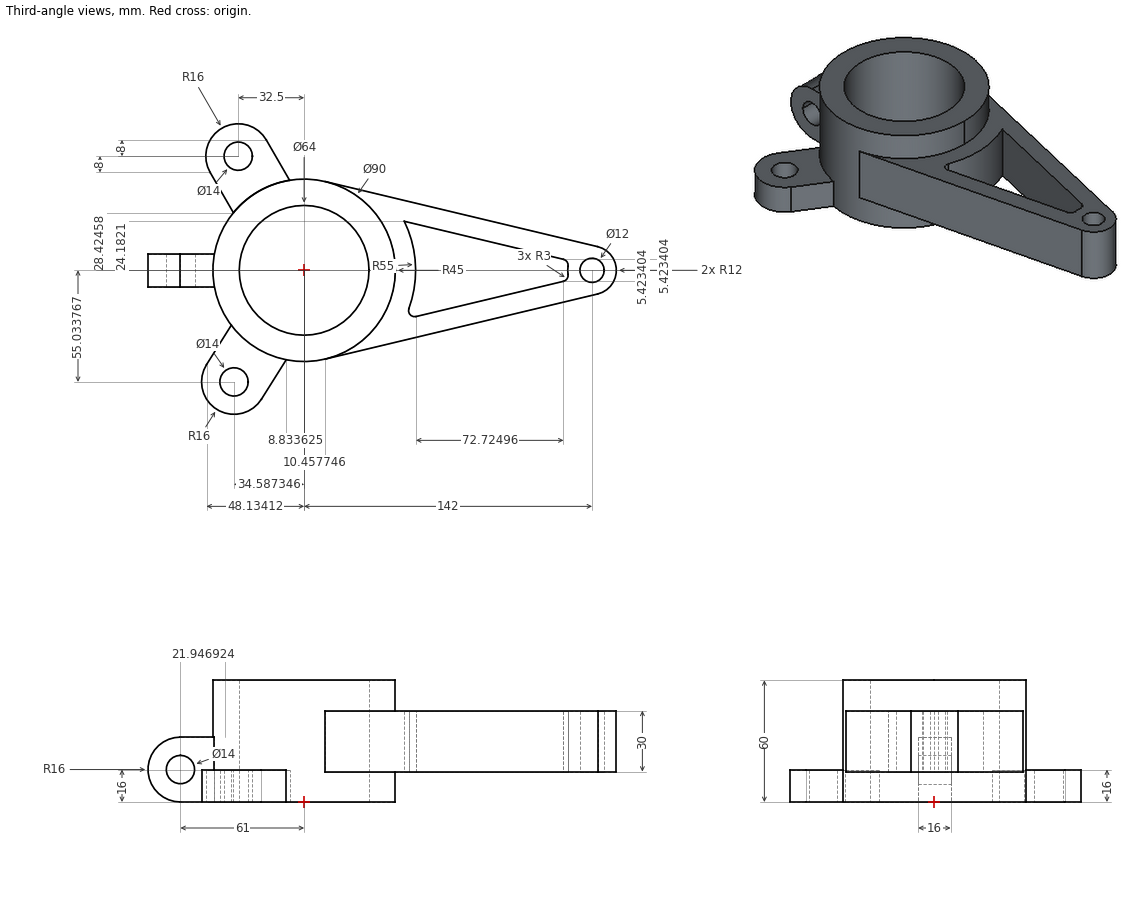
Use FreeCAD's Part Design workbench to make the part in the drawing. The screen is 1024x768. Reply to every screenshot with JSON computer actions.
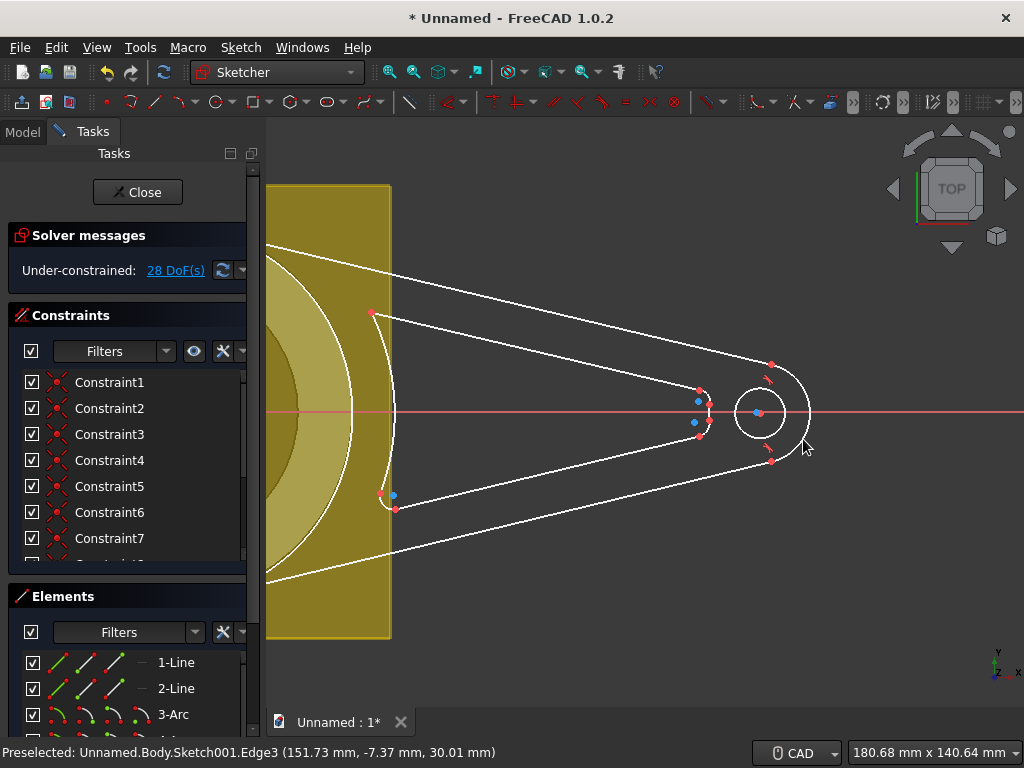
{"action": "left_click", "coordinate": [608, 458]}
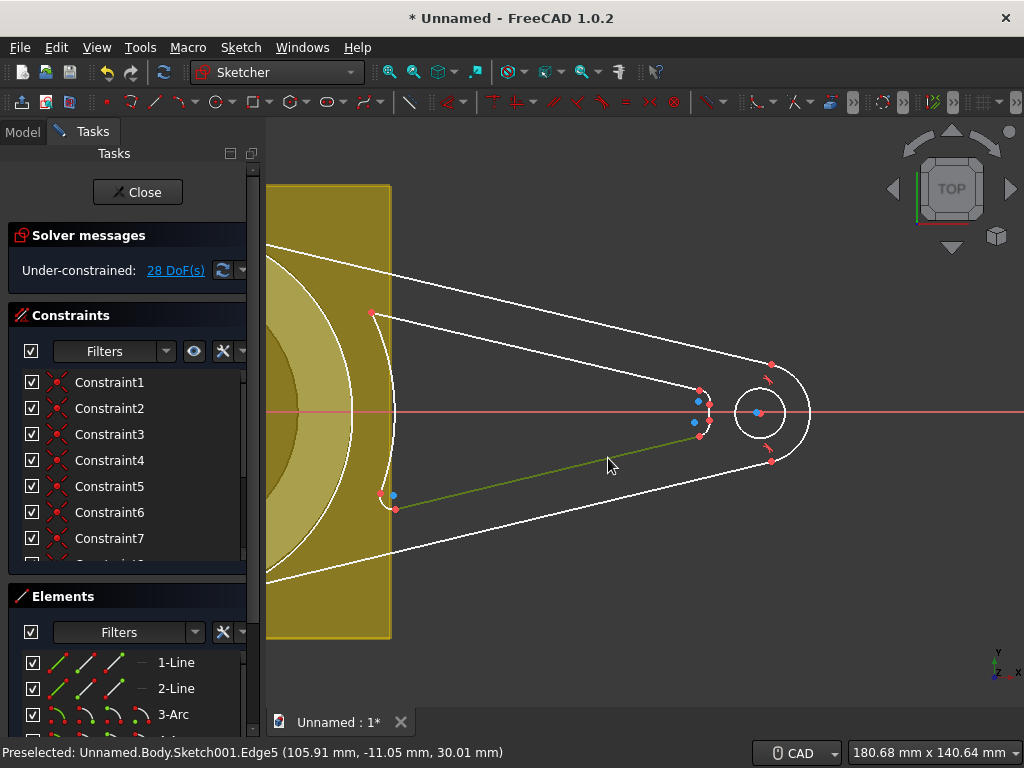
{"action": "left_click", "coordinate": [384, 505]}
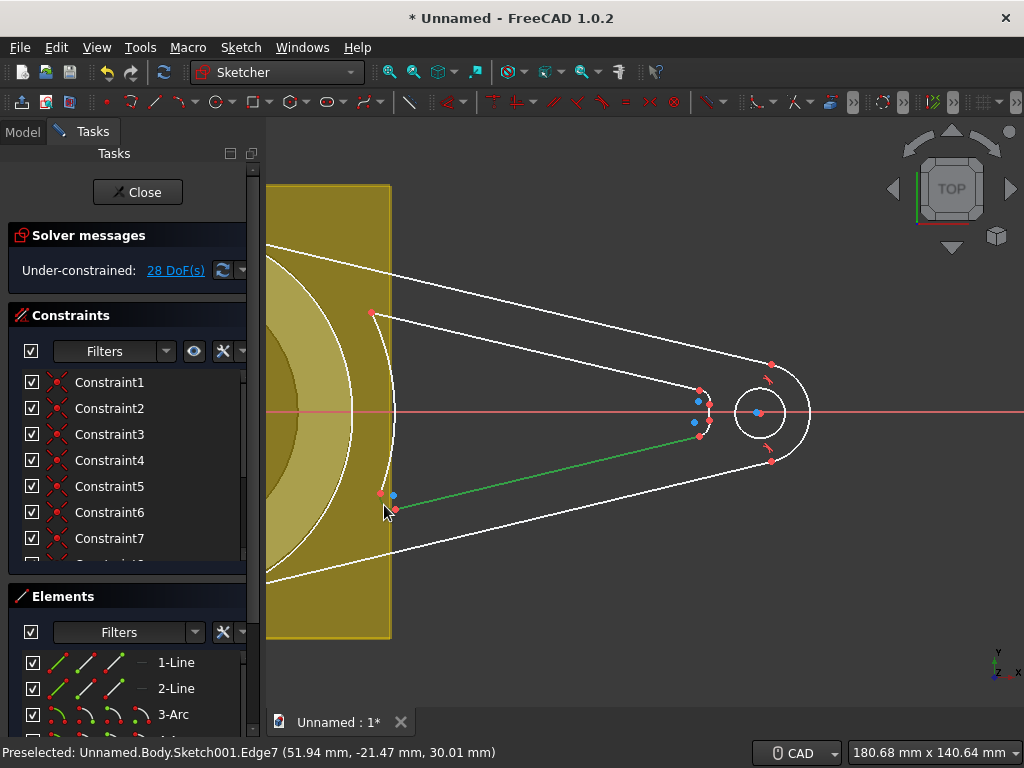
{"action": "key", "text": "t"}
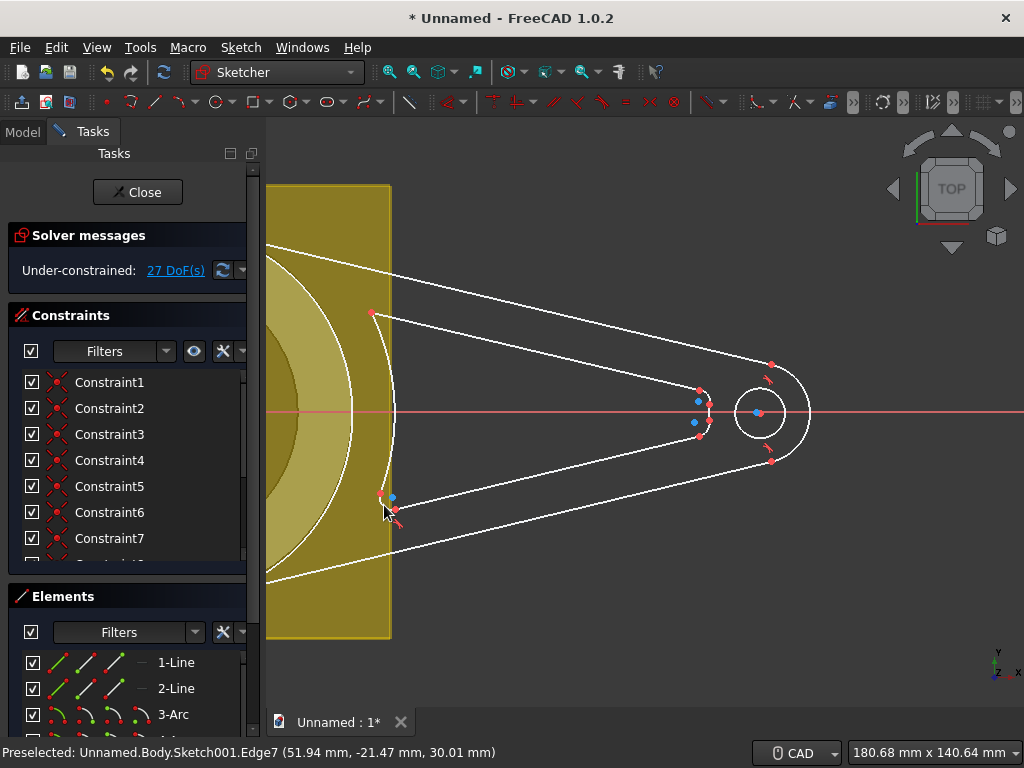
{"action": "left_click", "coordinate": [608, 458]}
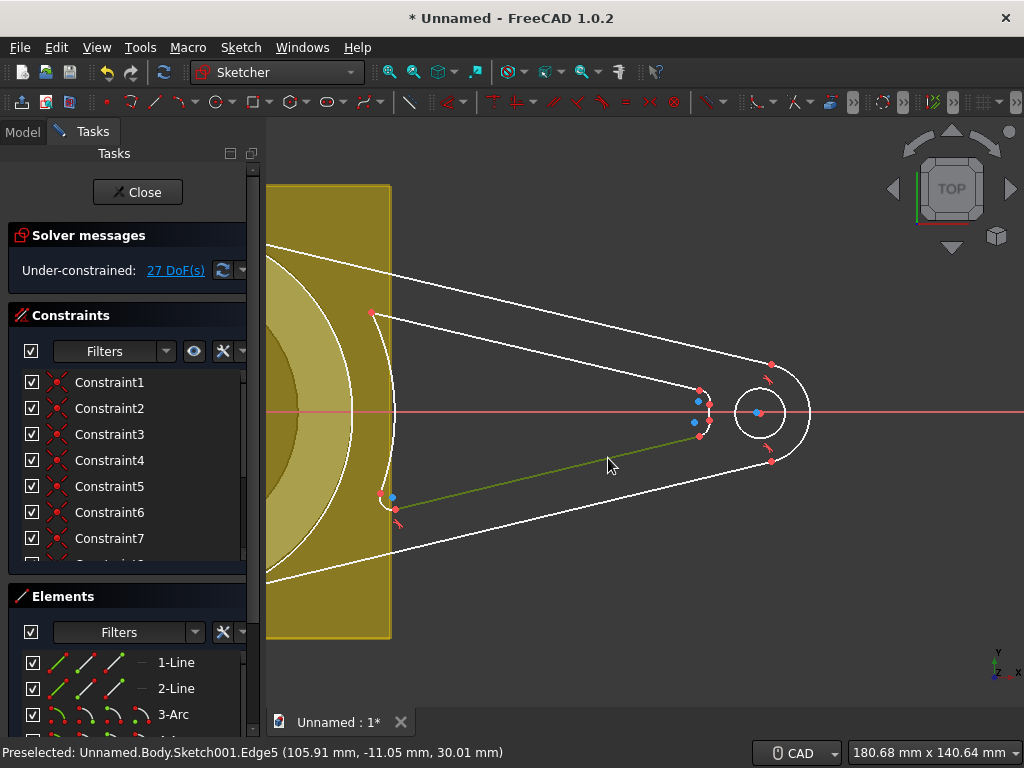
{"action": "scroll", "coordinate": [707, 430], "scroll_direction": "up", "scroll_amount": 2}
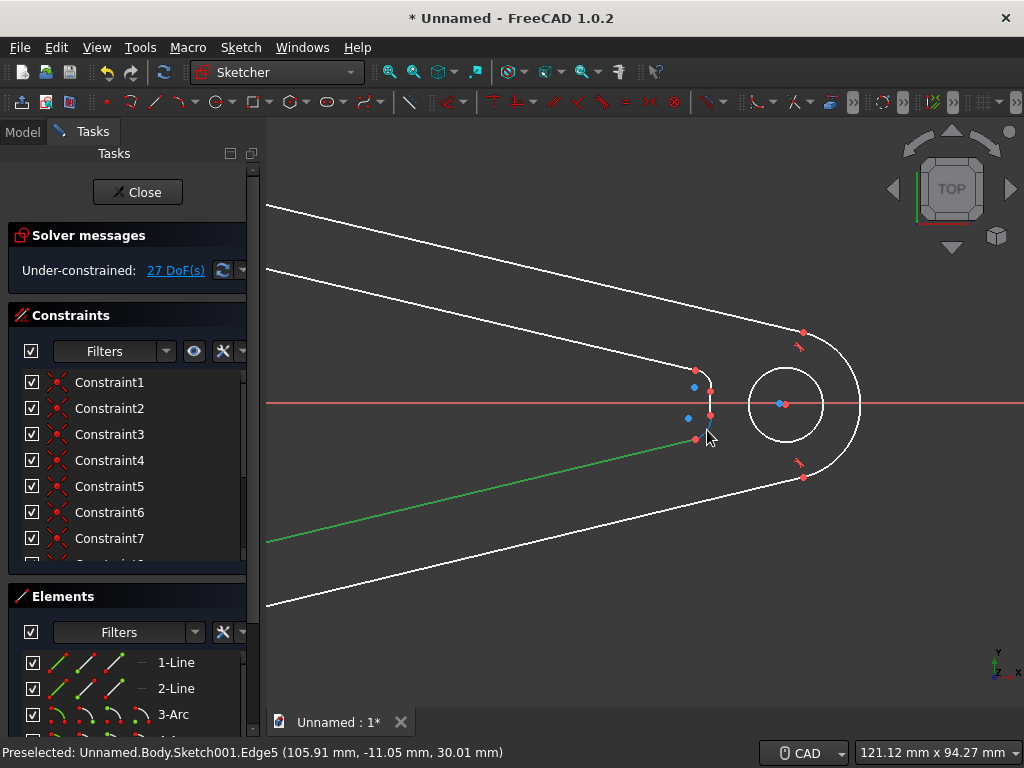
{"action": "left_click", "coordinate": [707, 430]}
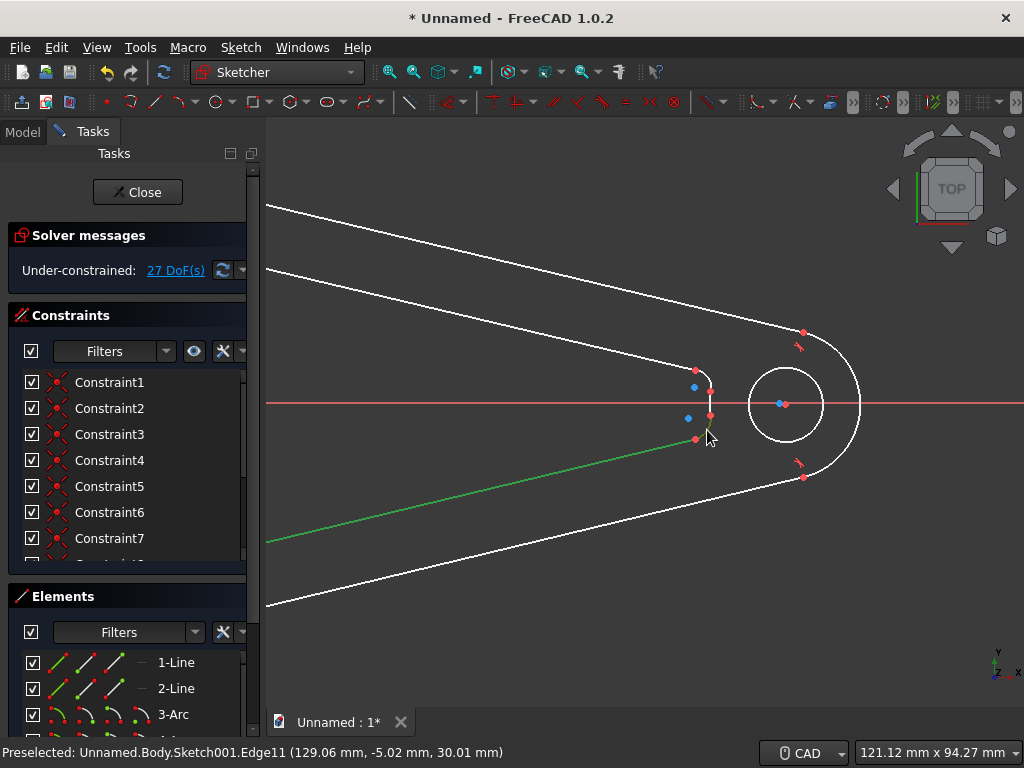
{"action": "key", "text": "t"}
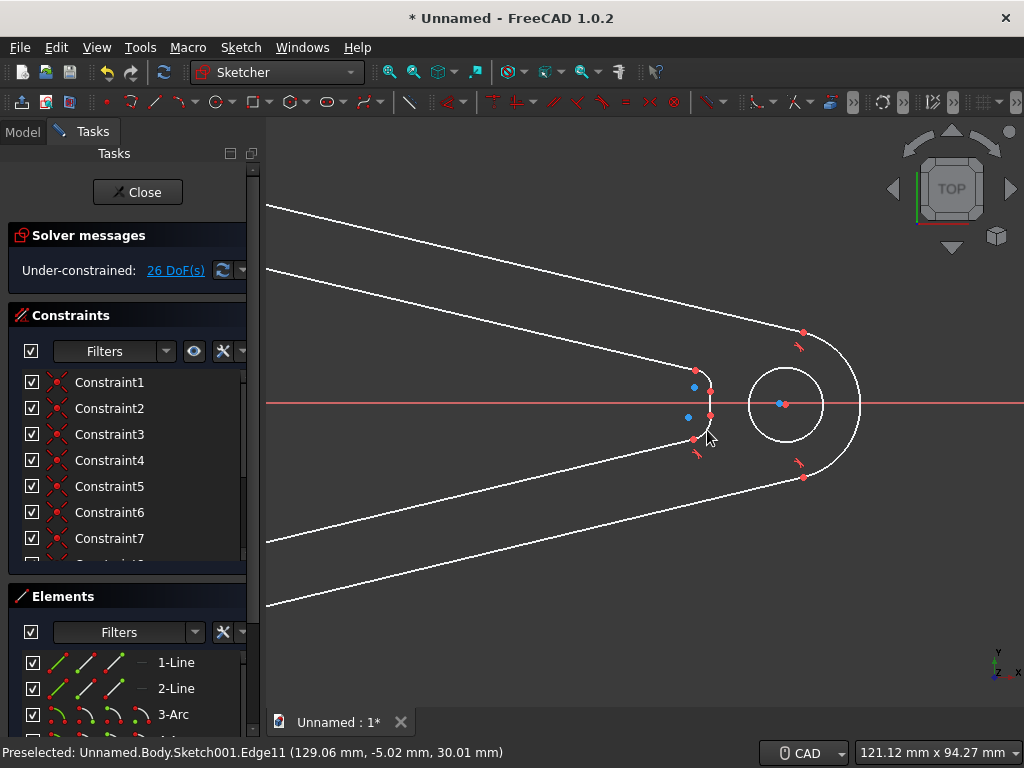
{"action": "left_click", "coordinate": [353, 289]}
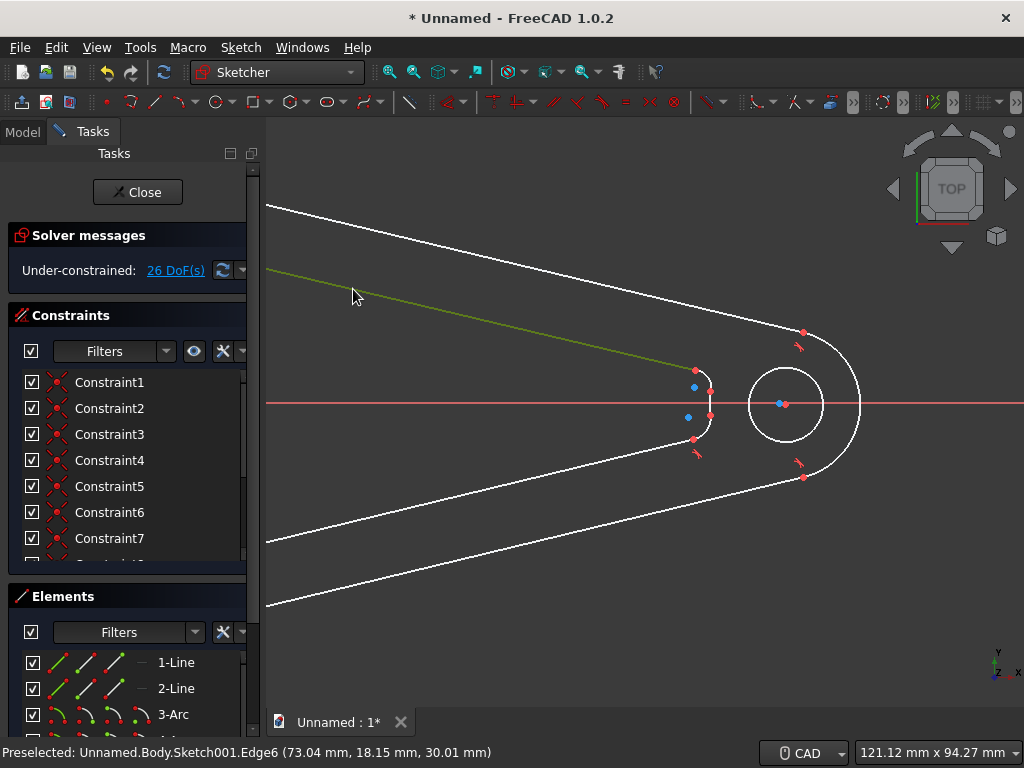
{"action": "left_click", "coordinate": [708, 377]}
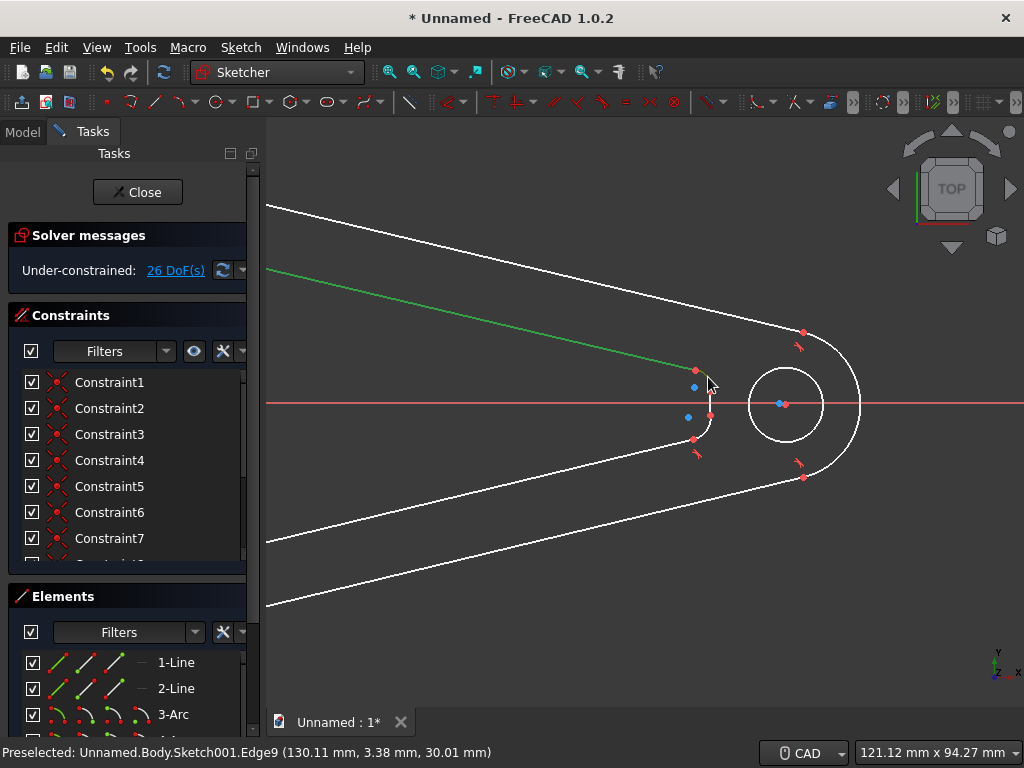
{"action": "key", "text": "t"}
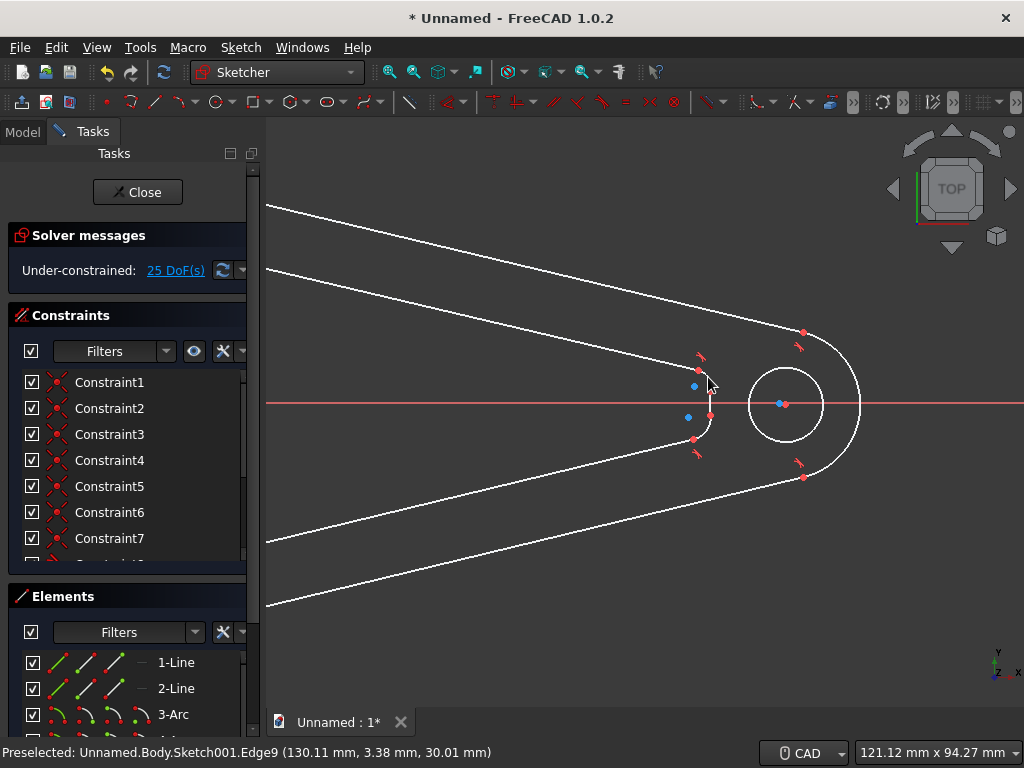
{"action": "scroll", "coordinate": [739, 419], "scroll_direction": "down", "scroll_amount": 4}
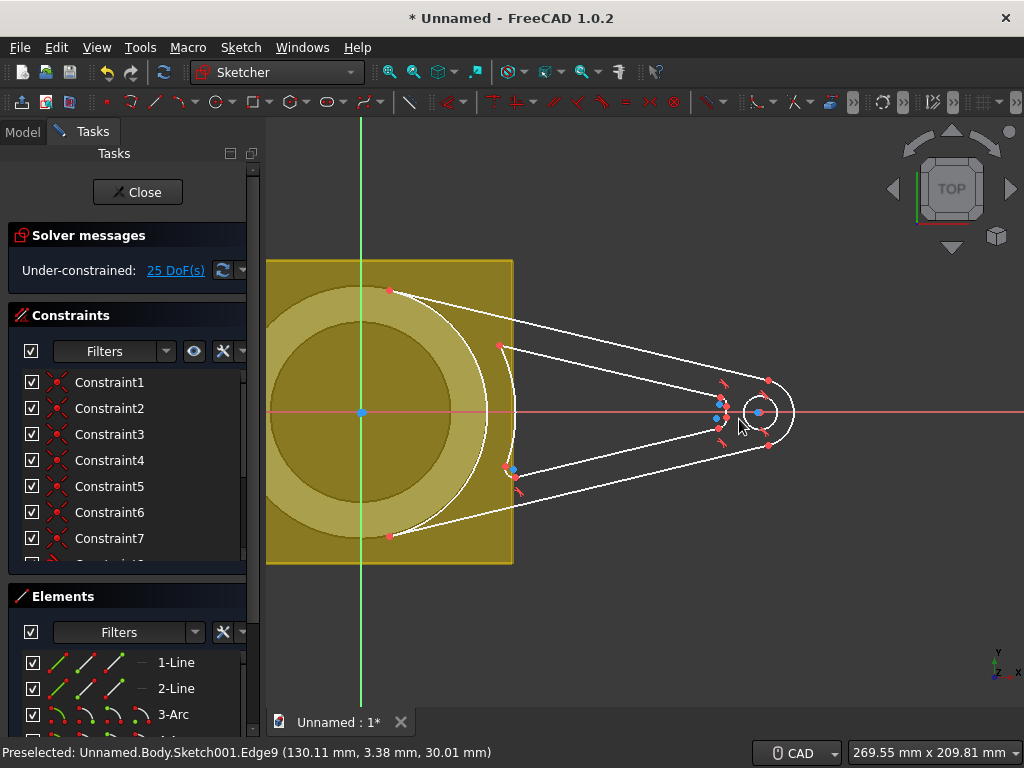
{"action": "scroll", "coordinate": [506, 472], "scroll_direction": "up", "scroll_amount": 5}